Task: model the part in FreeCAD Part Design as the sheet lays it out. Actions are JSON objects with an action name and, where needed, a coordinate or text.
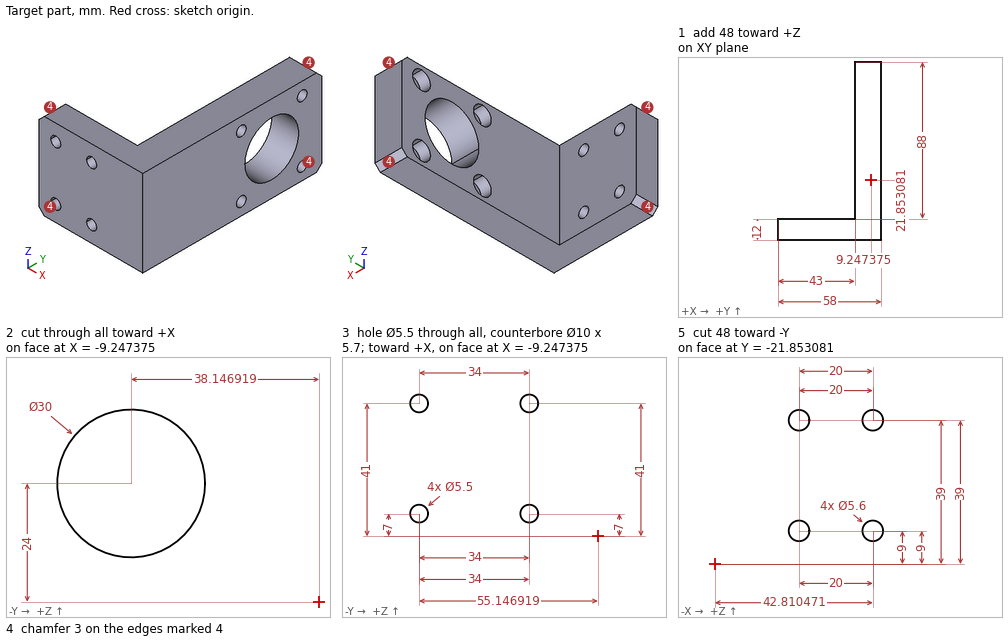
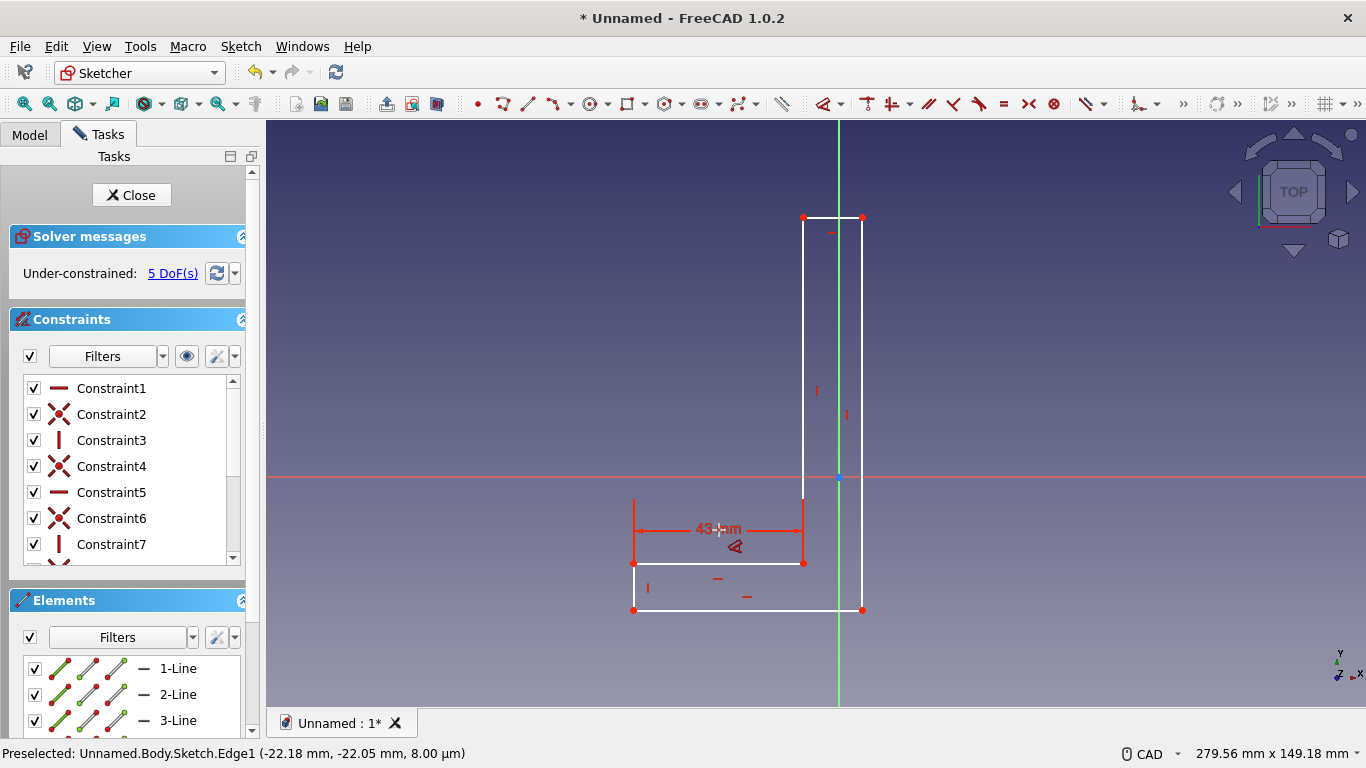
{"action": "left_click", "coordinate": [634, 578]}
{"action": "left_click", "coordinate": [600, 587]}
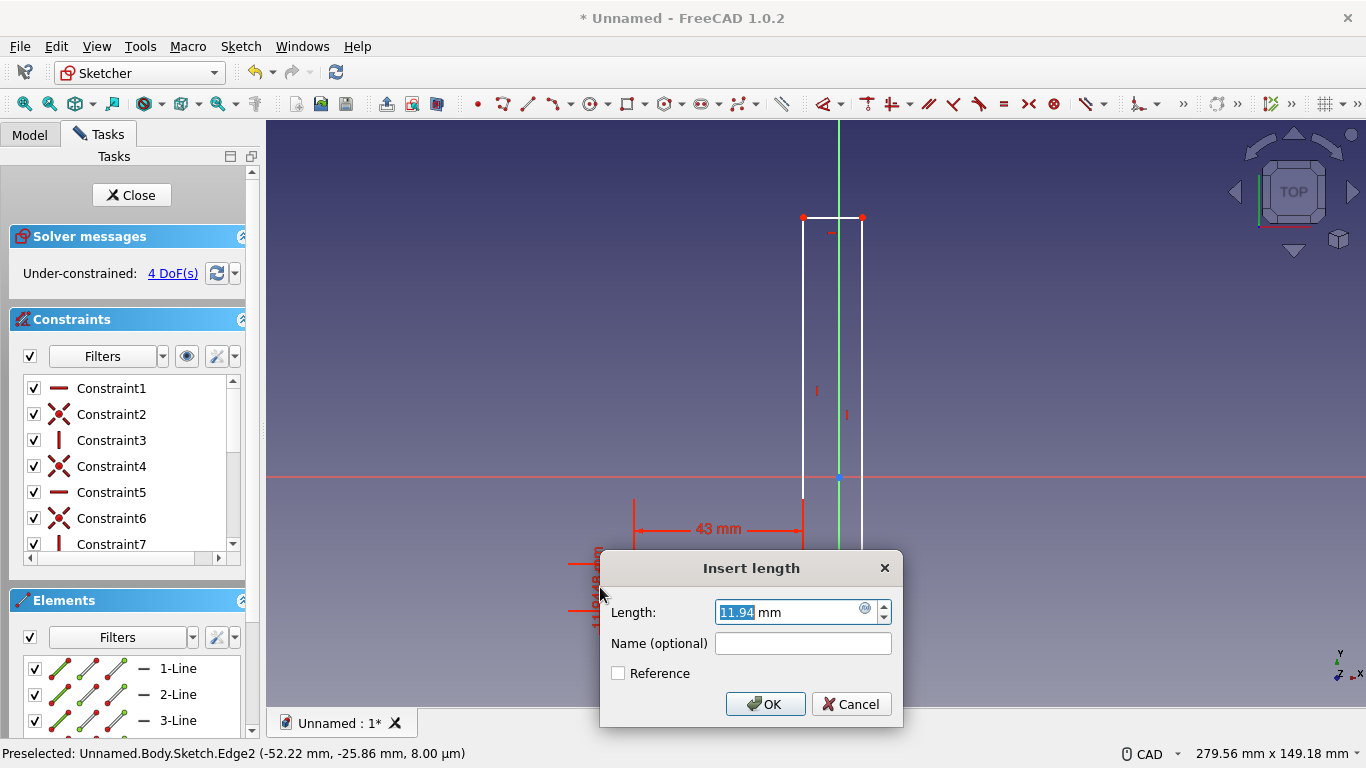
{"action": "type", "text": "12"}
{"action": "key", "text": "Return"}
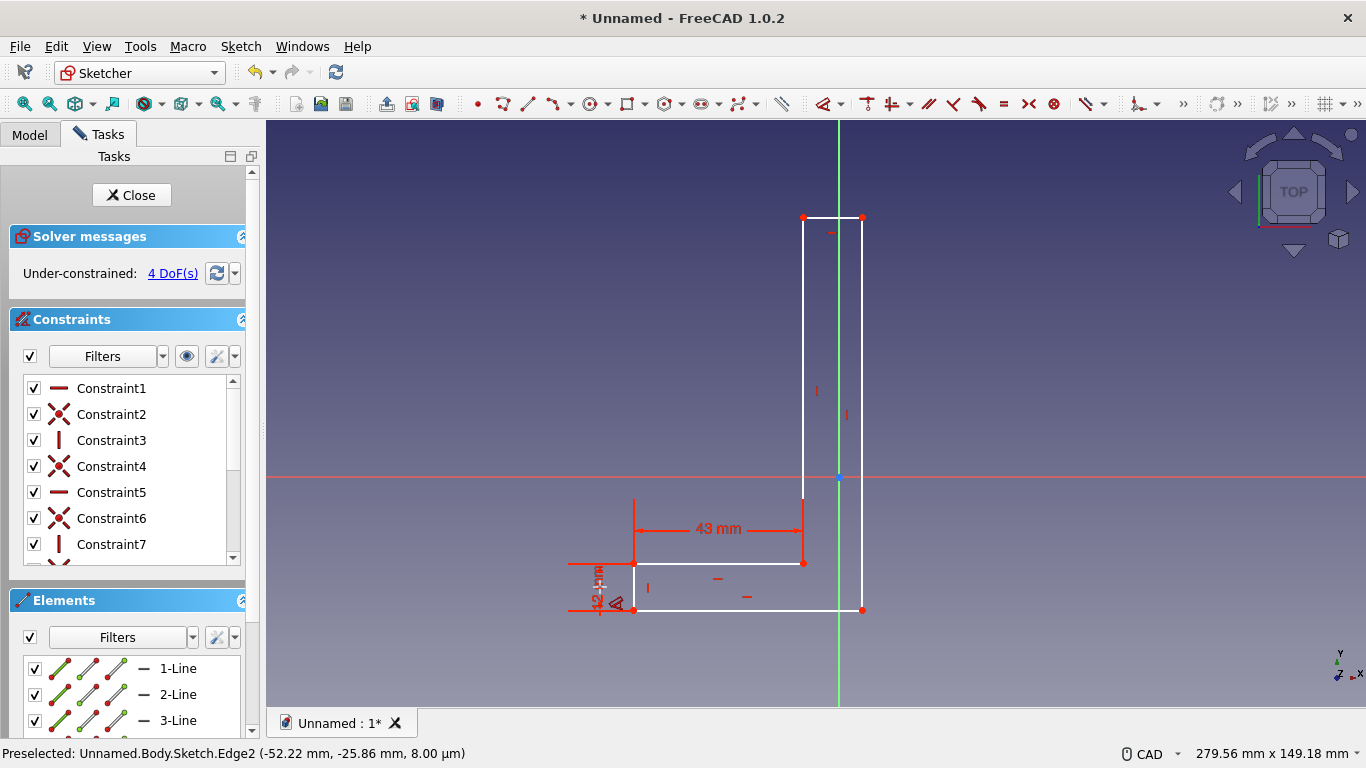
{"action": "left_click", "coordinate": [702, 611]}
{"action": "left_click", "coordinate": [748, 645]}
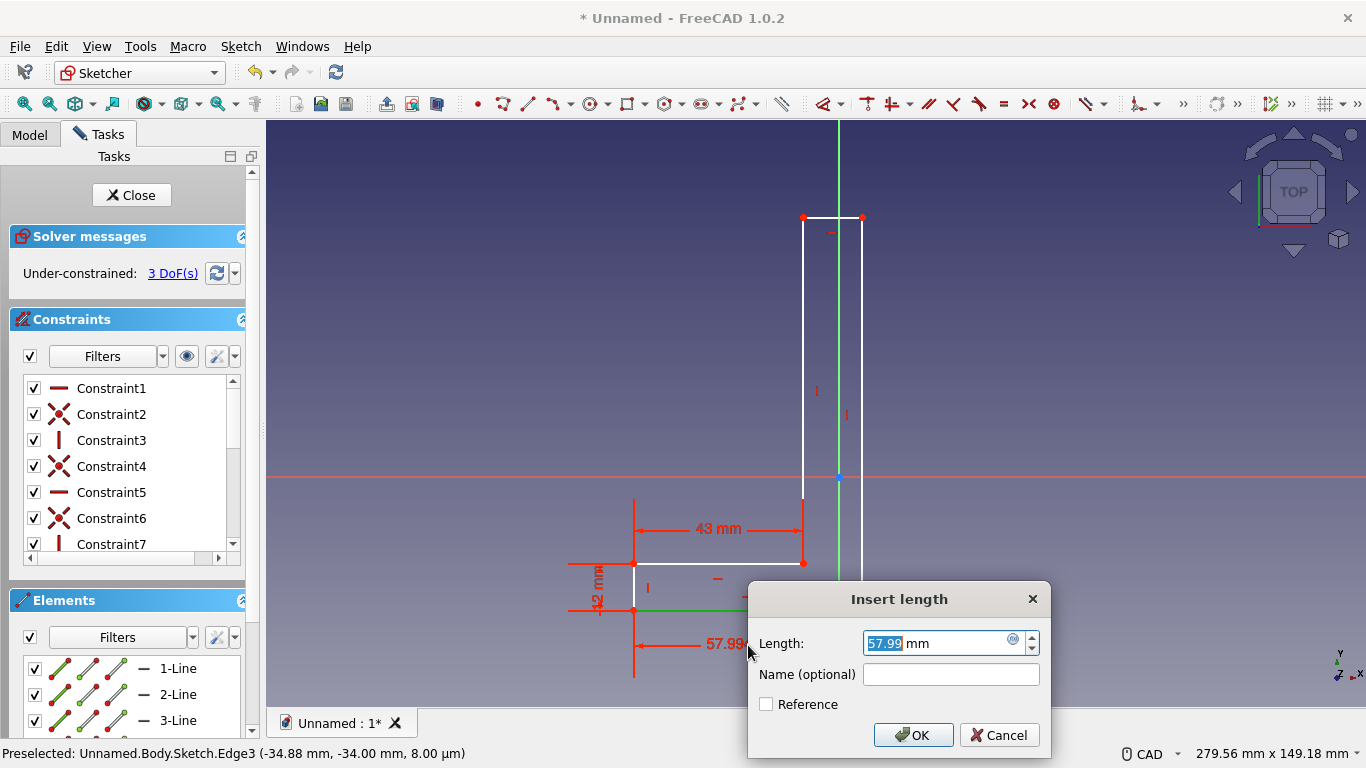
{"action": "type", "text": "58"}
{"action": "key", "text": "Return"}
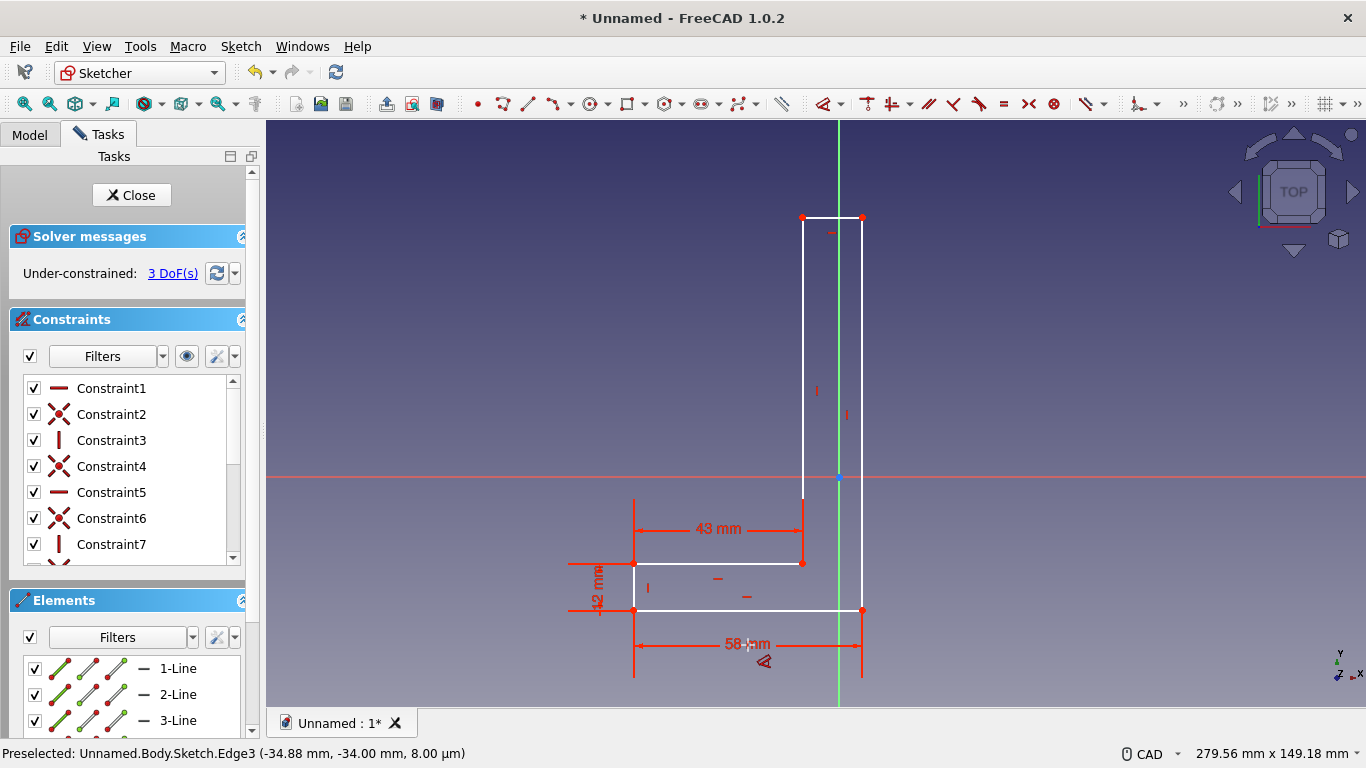
{"action": "left_click", "coordinate": [803, 322]}
{"action": "left_click", "coordinate": [769, 391]}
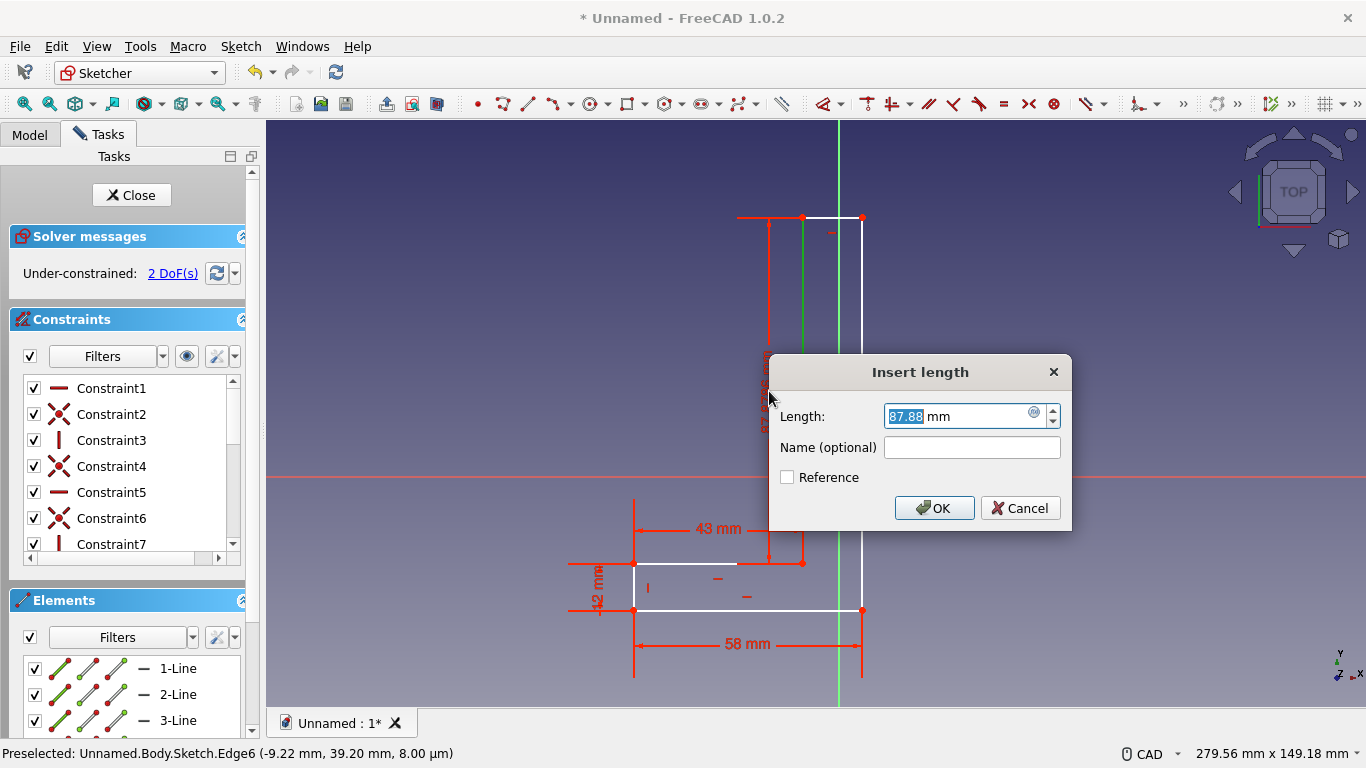
{"action": "type", "text": "88"}
{"action": "key", "text": "Return"}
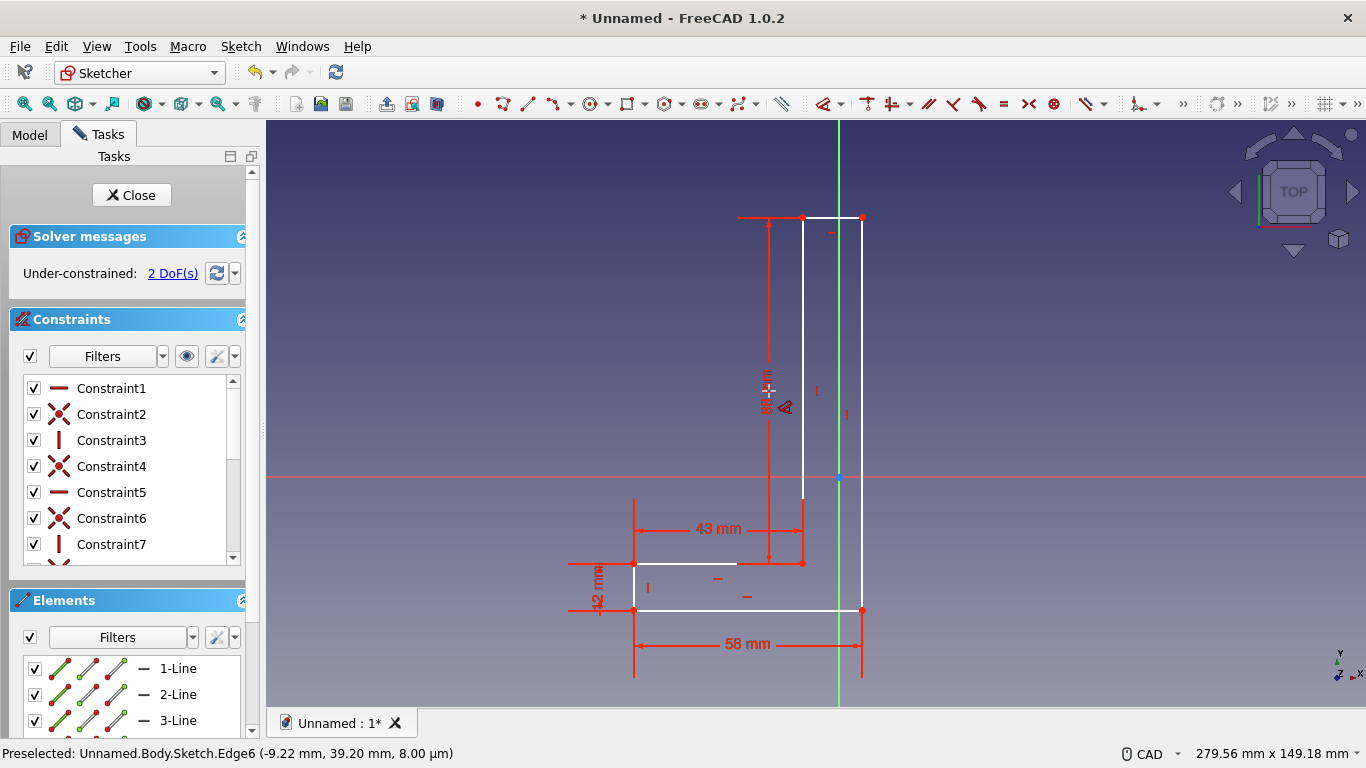
{"action": "left_click", "coordinate": [803, 564]}
{"action": "left_click", "coordinate": [821, 598]}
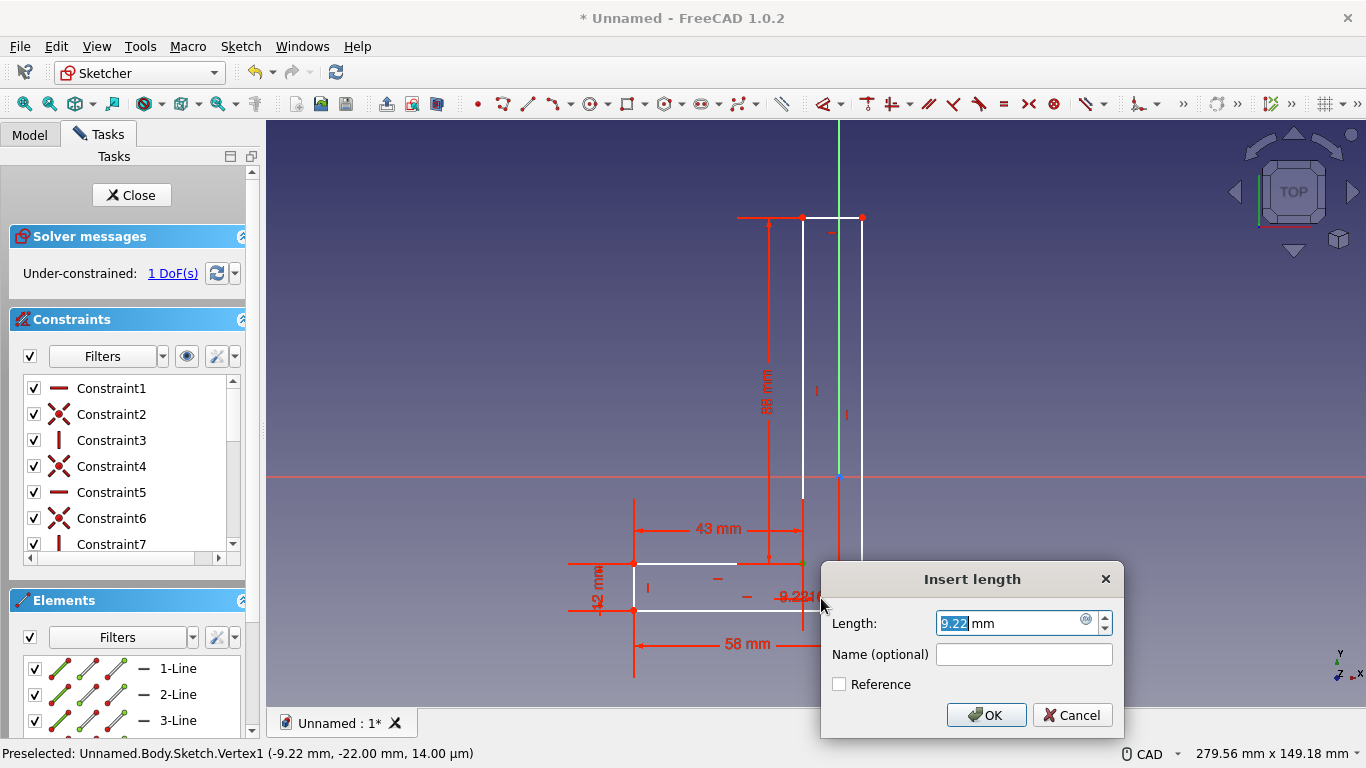
{"action": "type", "text": "9.247375"}
{"action": "key", "text": "Return"}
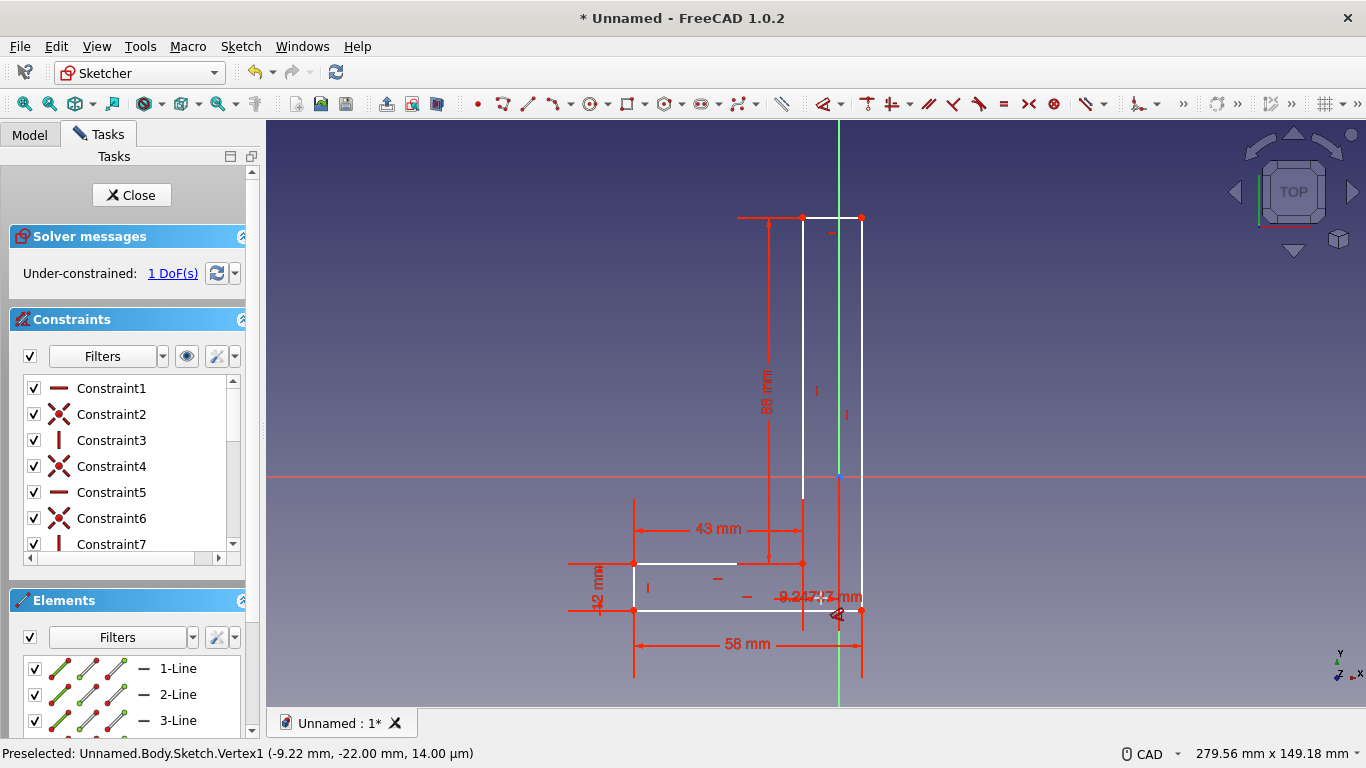
{"action": "left_click", "coordinate": [803, 564]}
{"action": "left_click", "coordinate": [769, 501]}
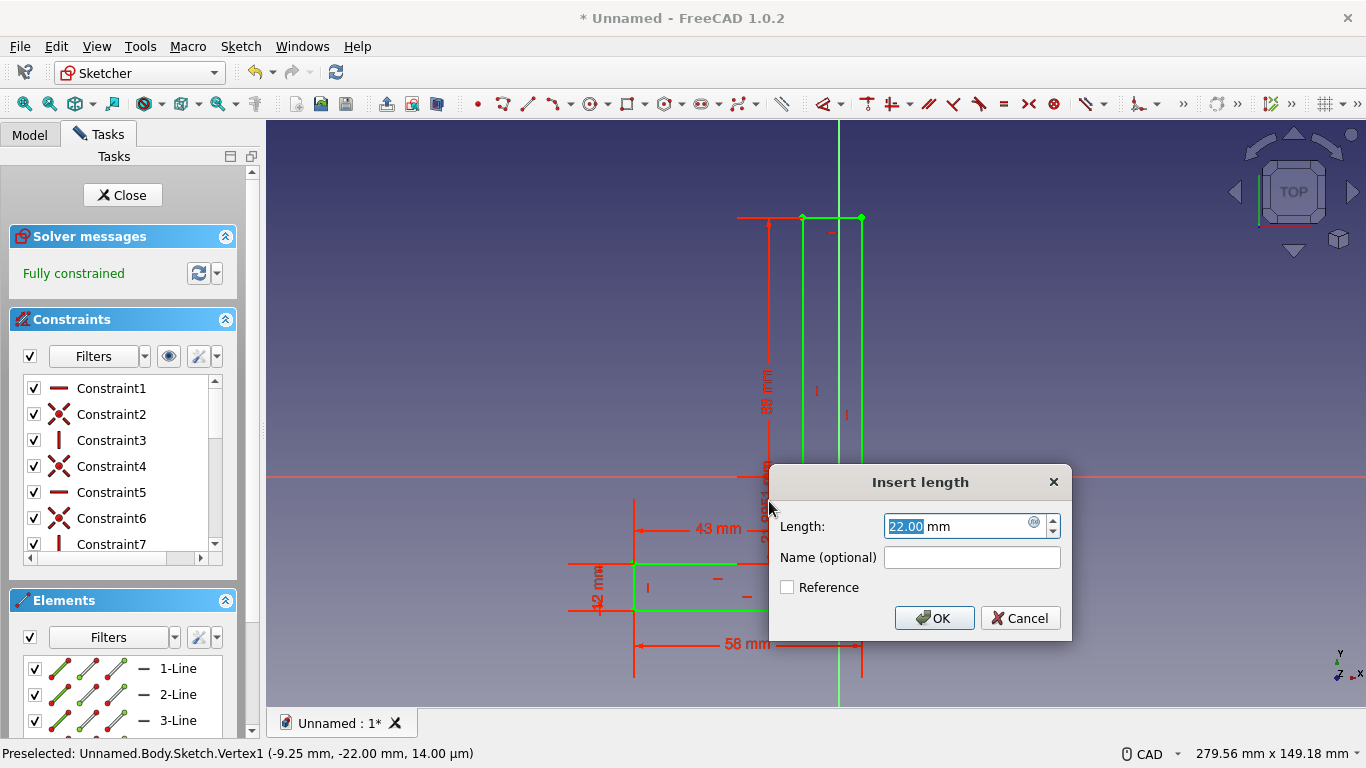
{"action": "type", "text": "21.853081"}
{"action": "key", "text": "Return"}
{"action": "key", "text": "Escape"}